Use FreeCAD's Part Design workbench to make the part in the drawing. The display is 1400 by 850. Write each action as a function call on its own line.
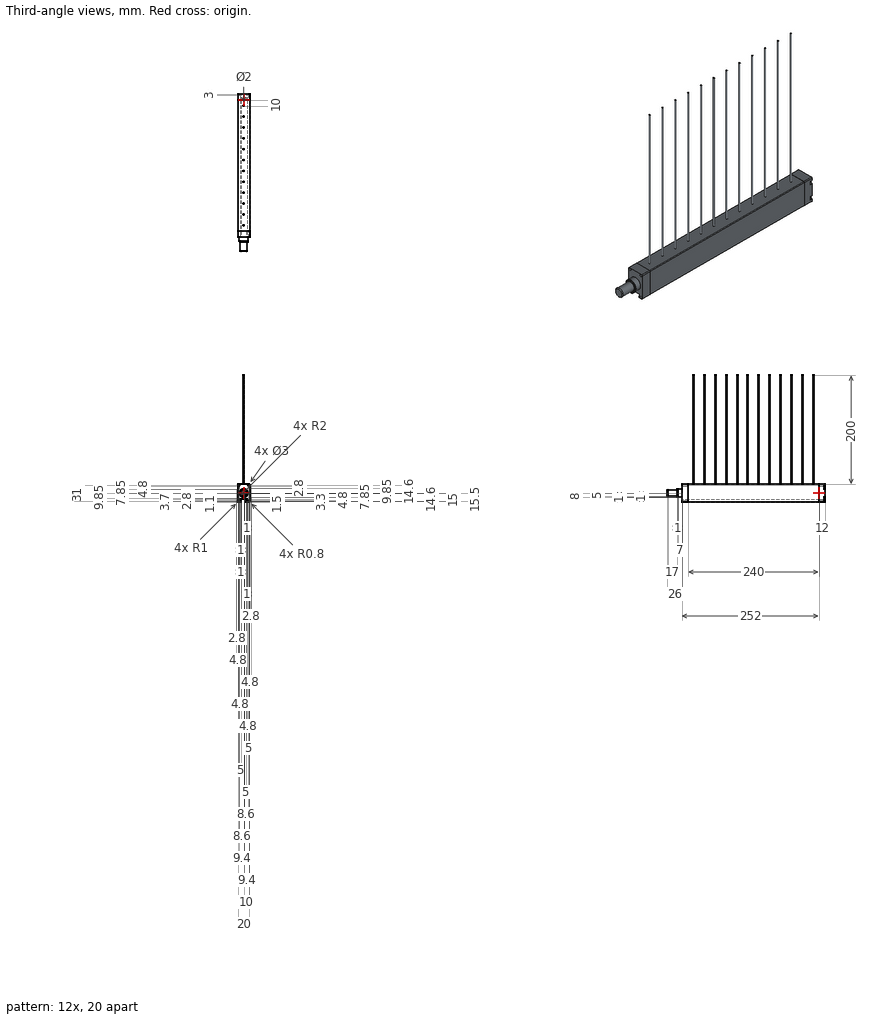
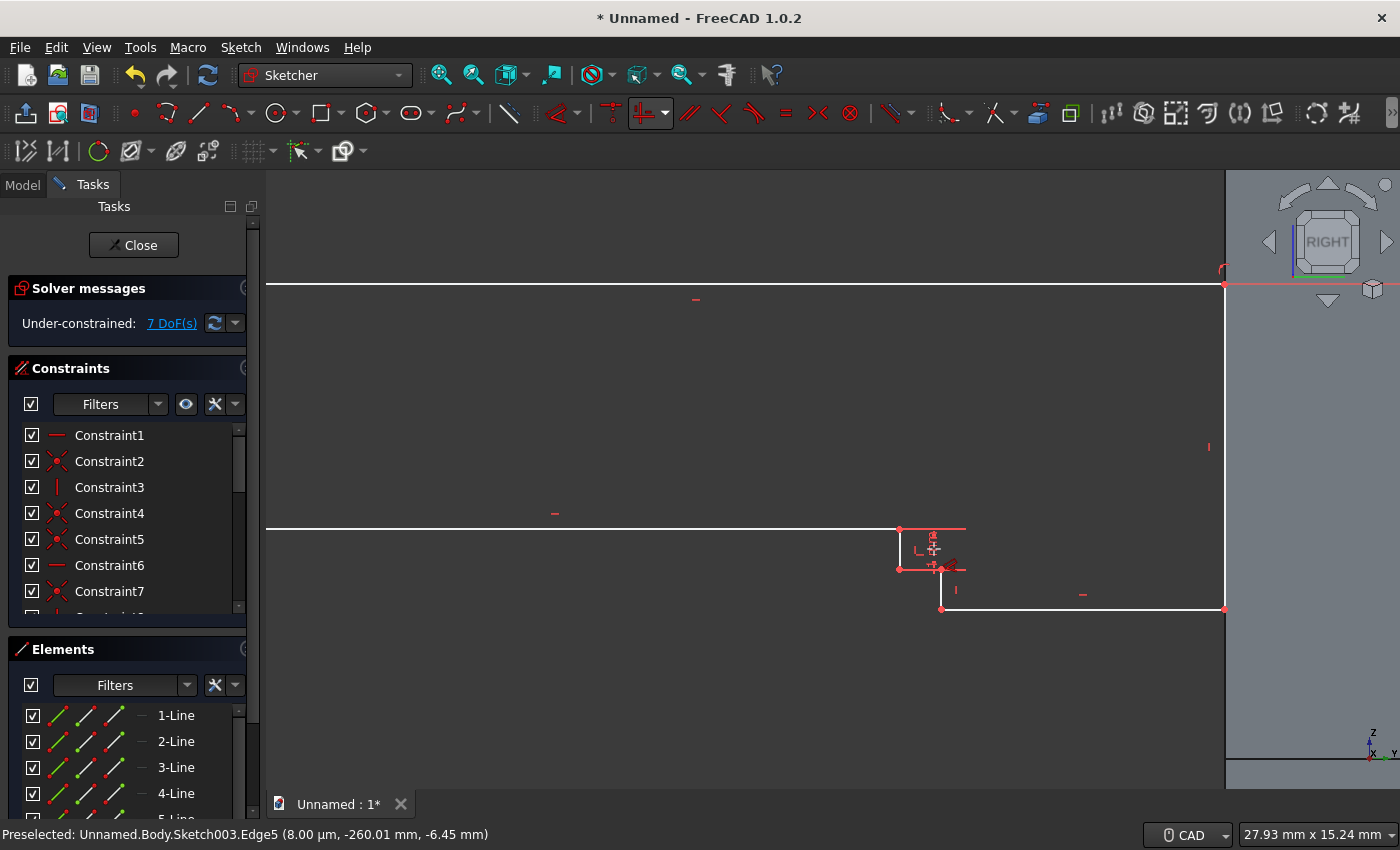
click(912, 570)
click(921, 604)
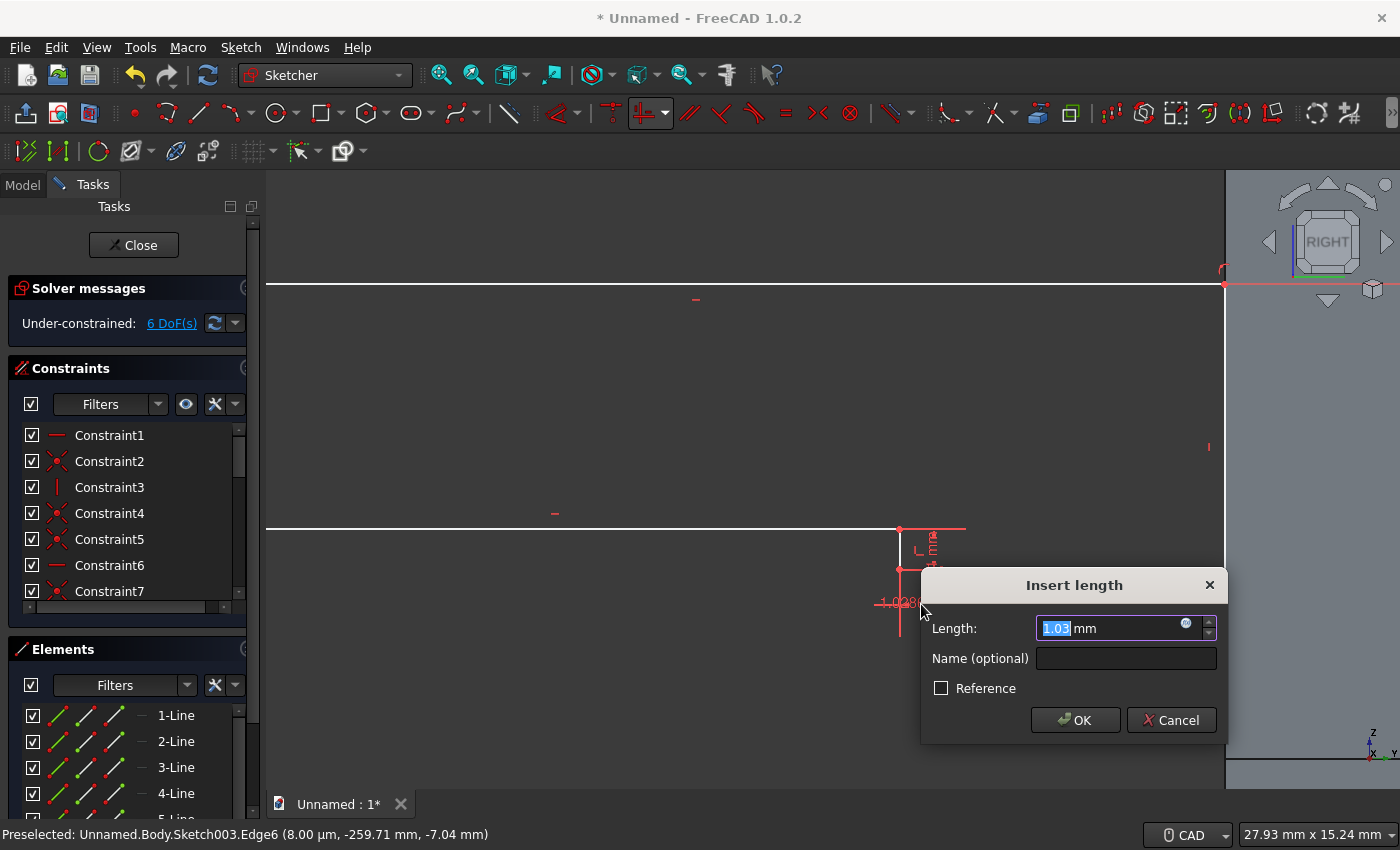
text(1)
key(Return)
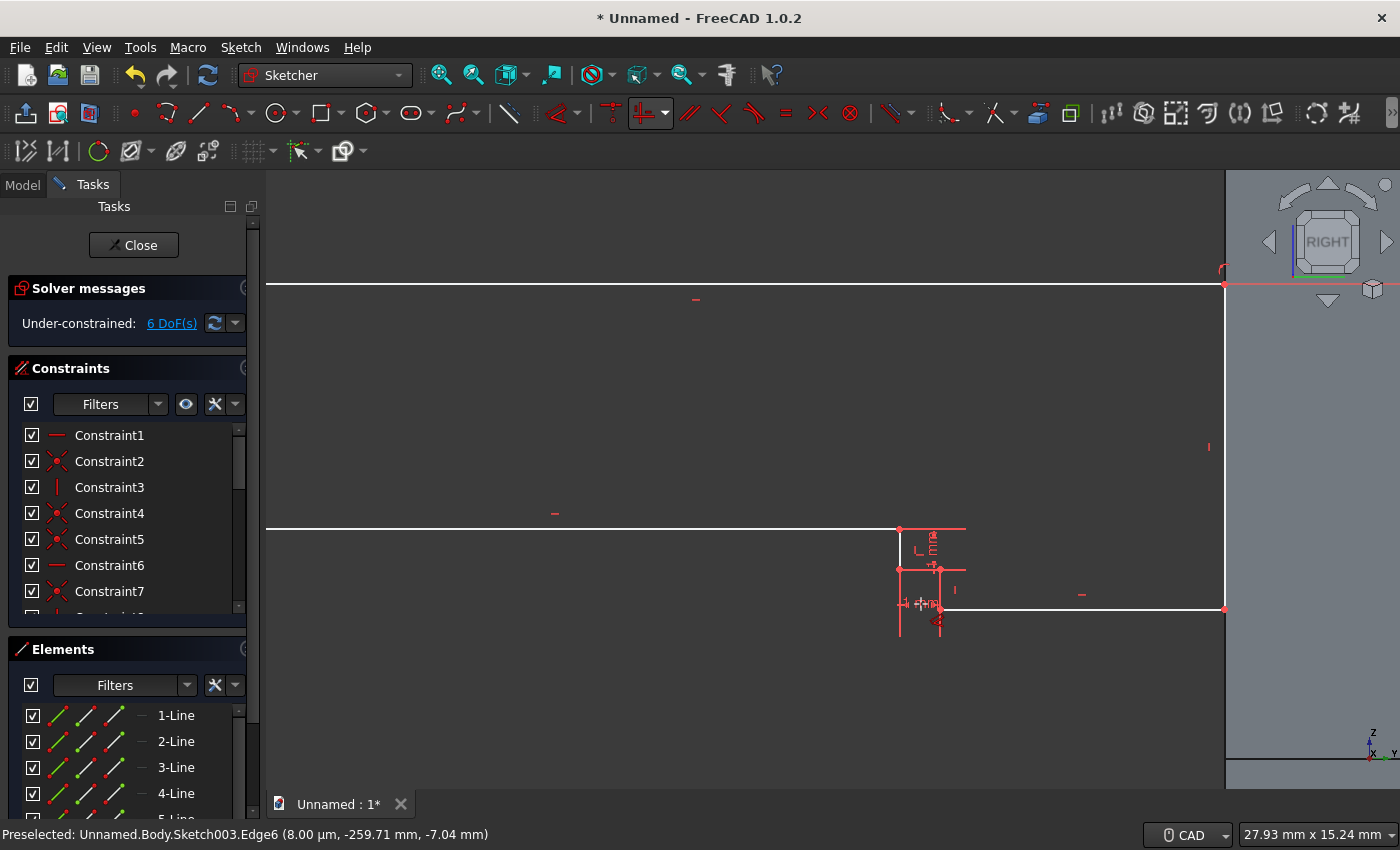
click(940, 582)
click(974, 581)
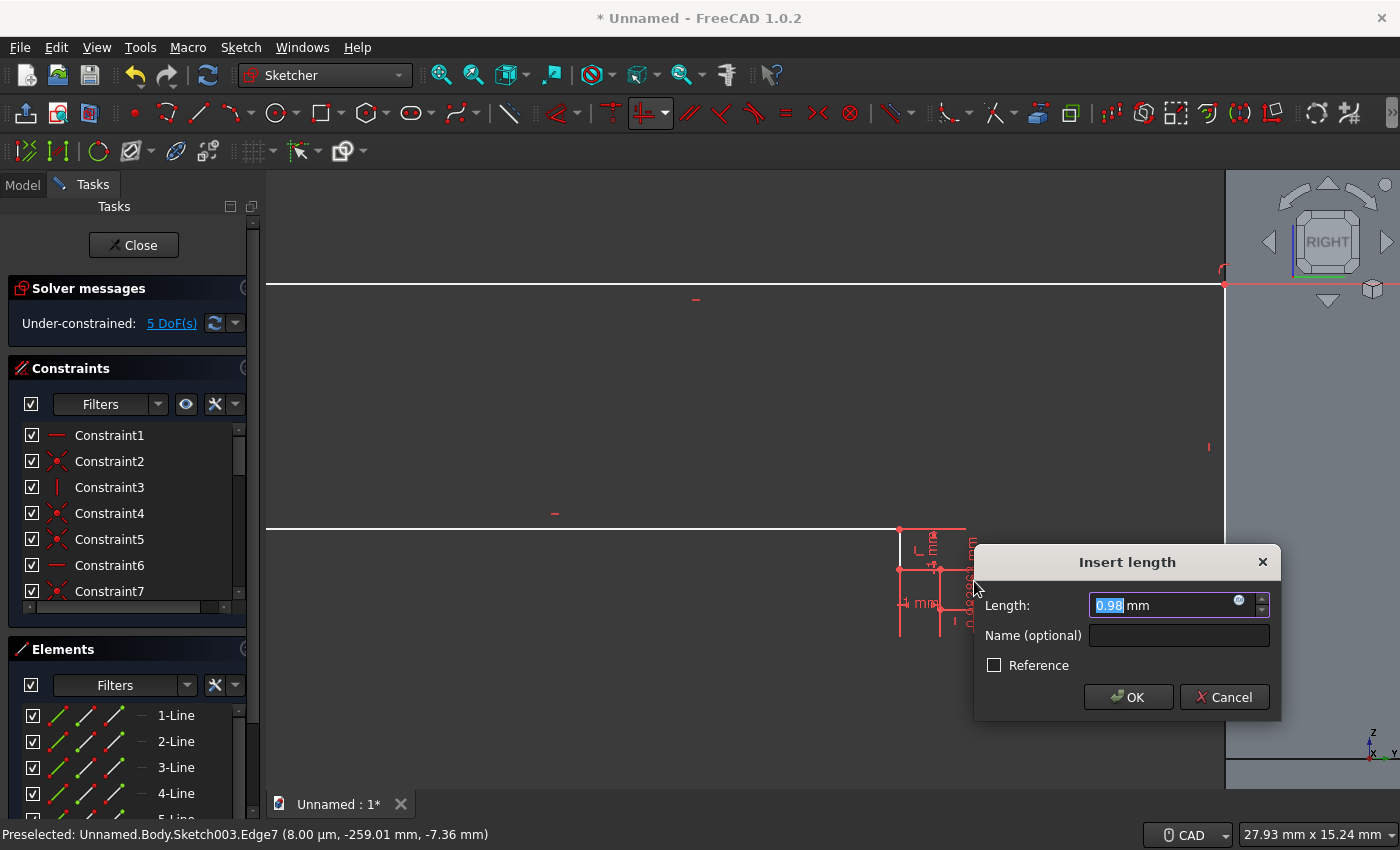
text(1)
key(Return)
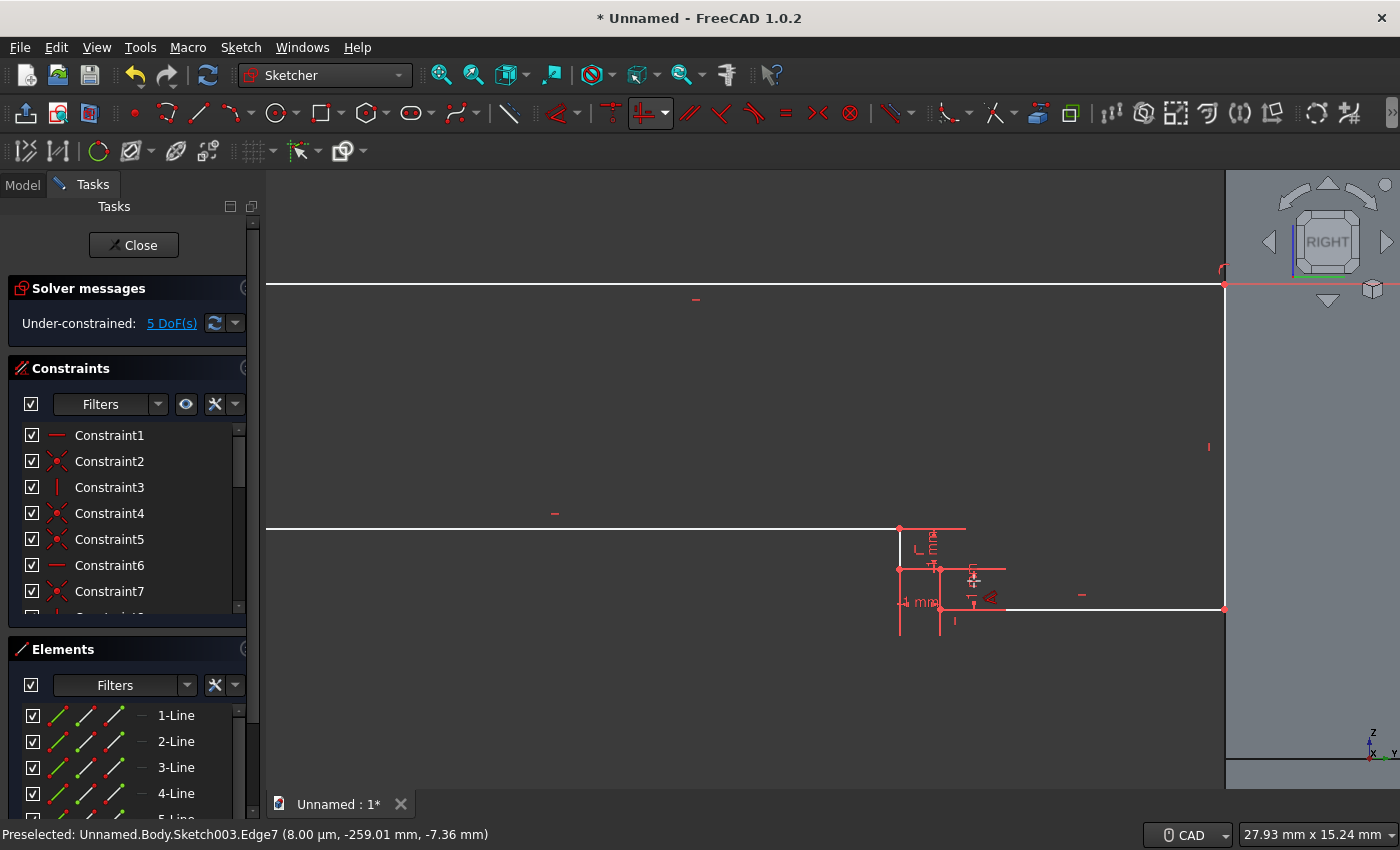
click(1026, 610)
click(1083, 644)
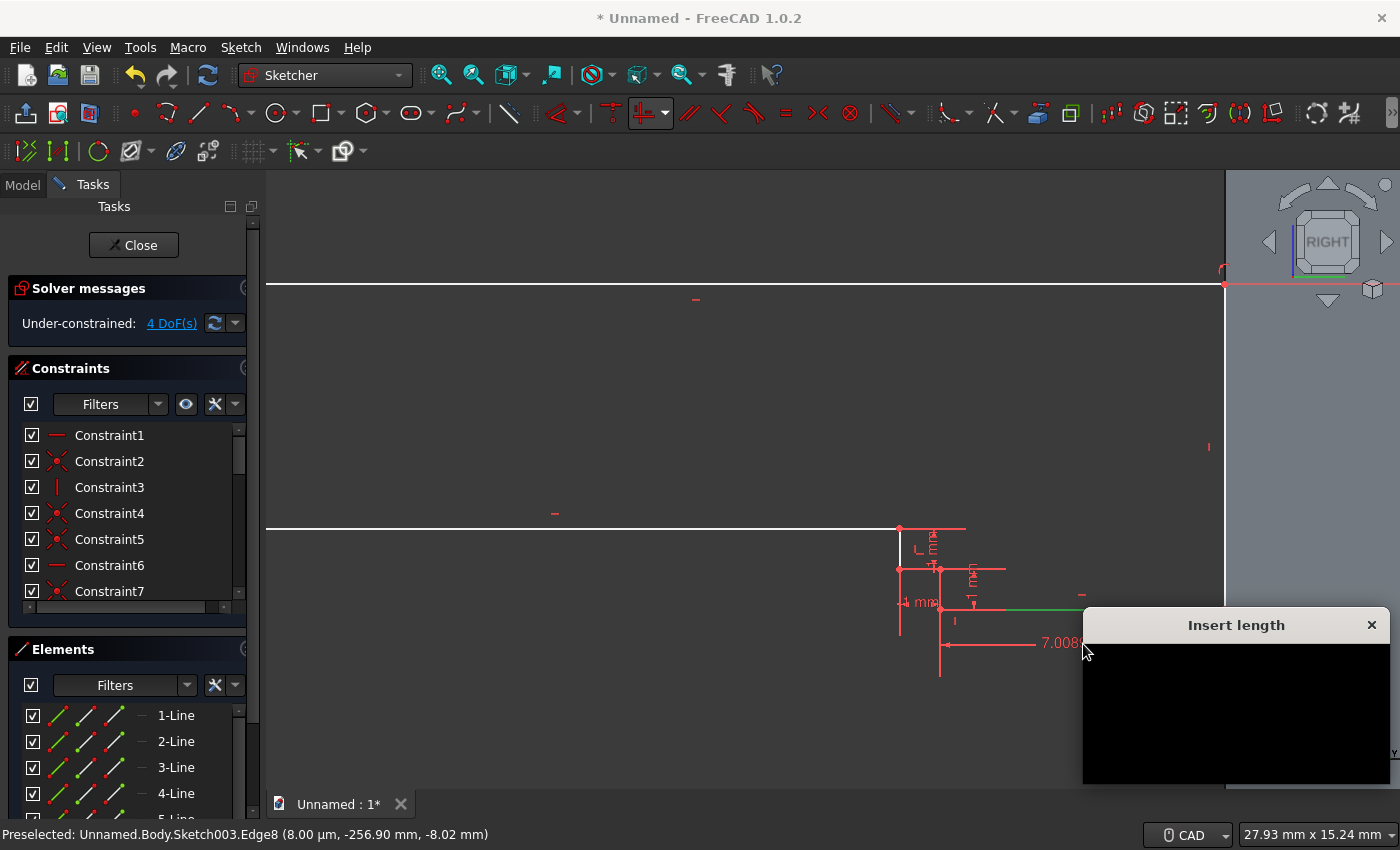
text(7)
key(Return)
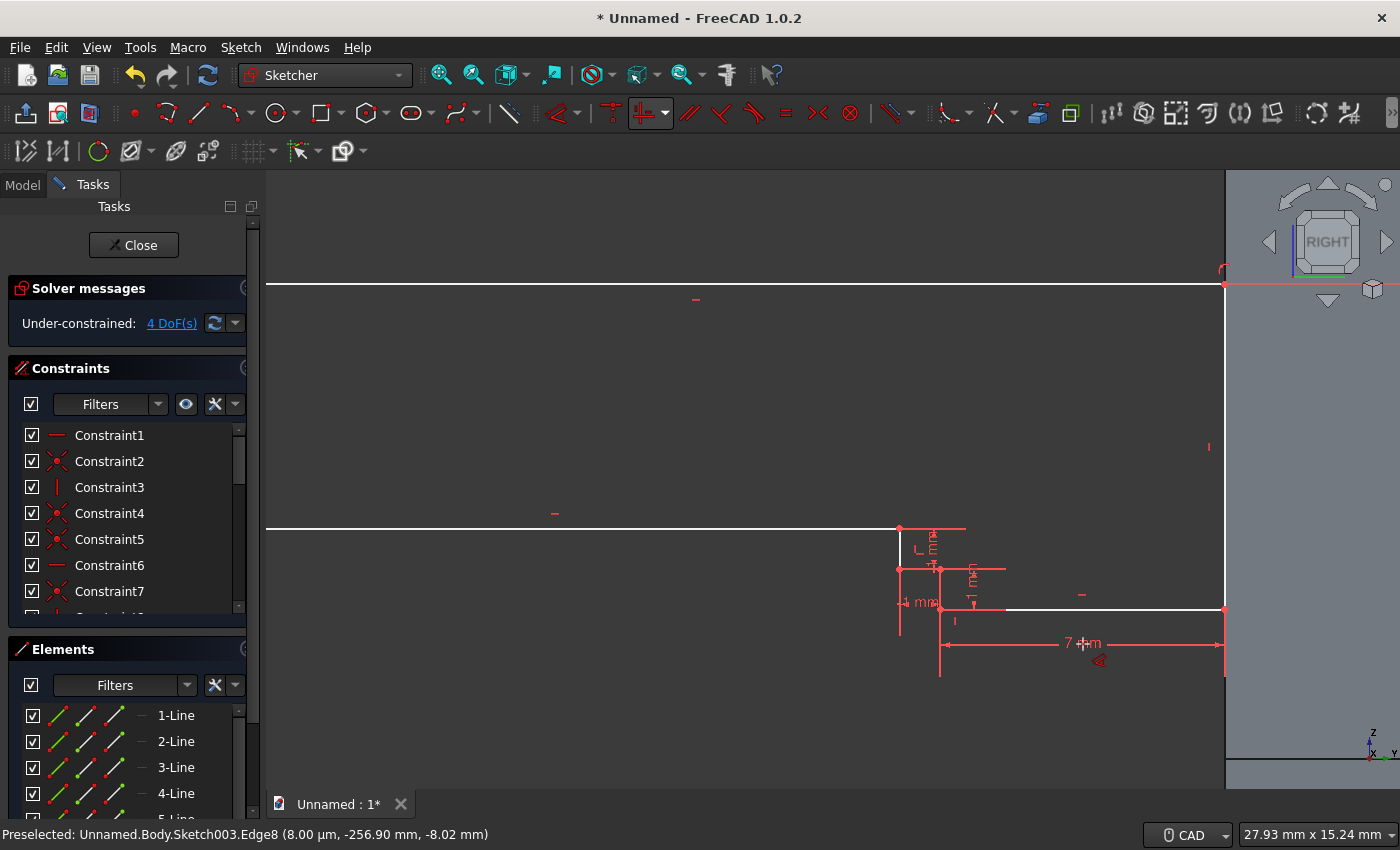
click(1225, 512)
click(1191, 447)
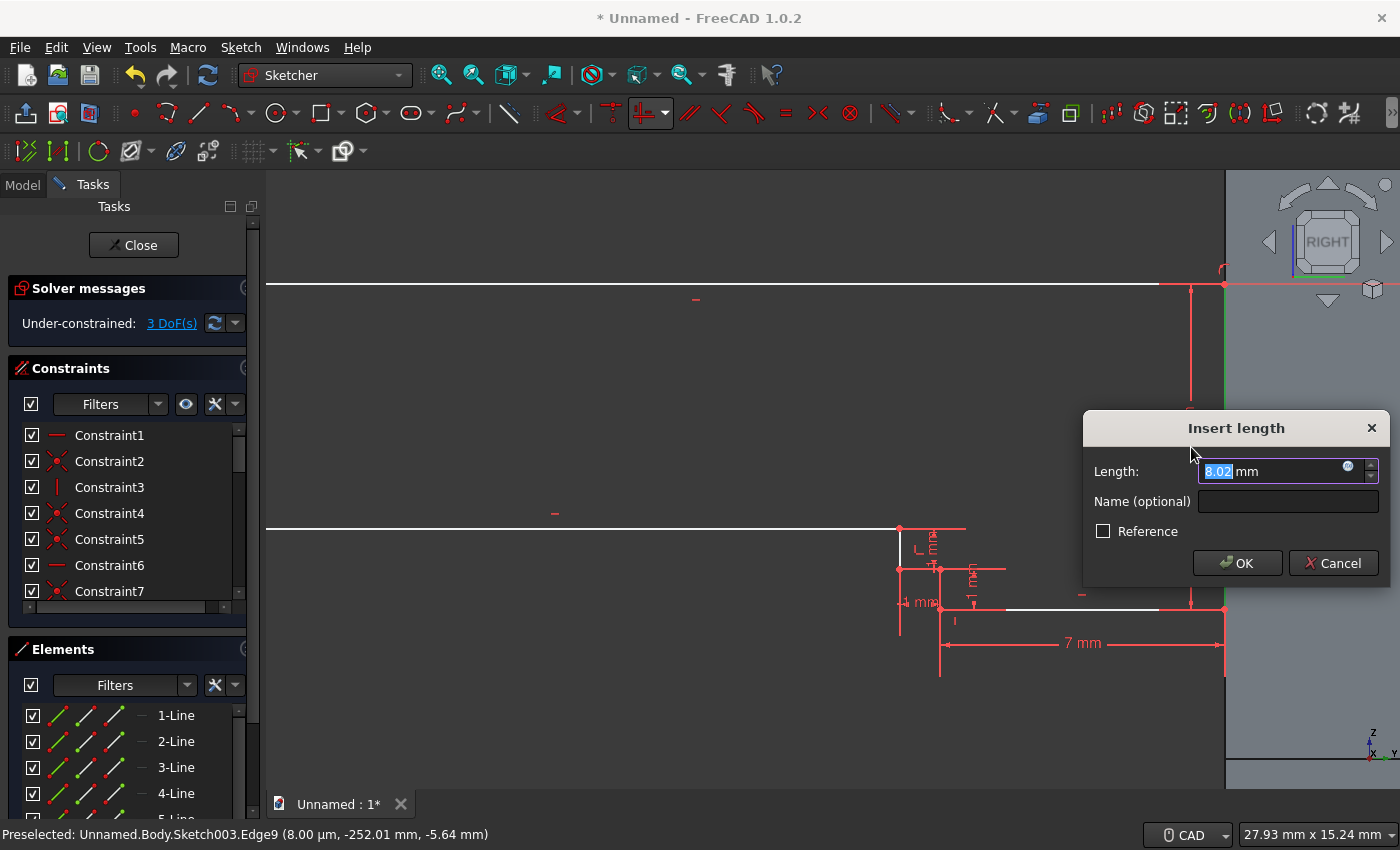
text(8)
key(Return)